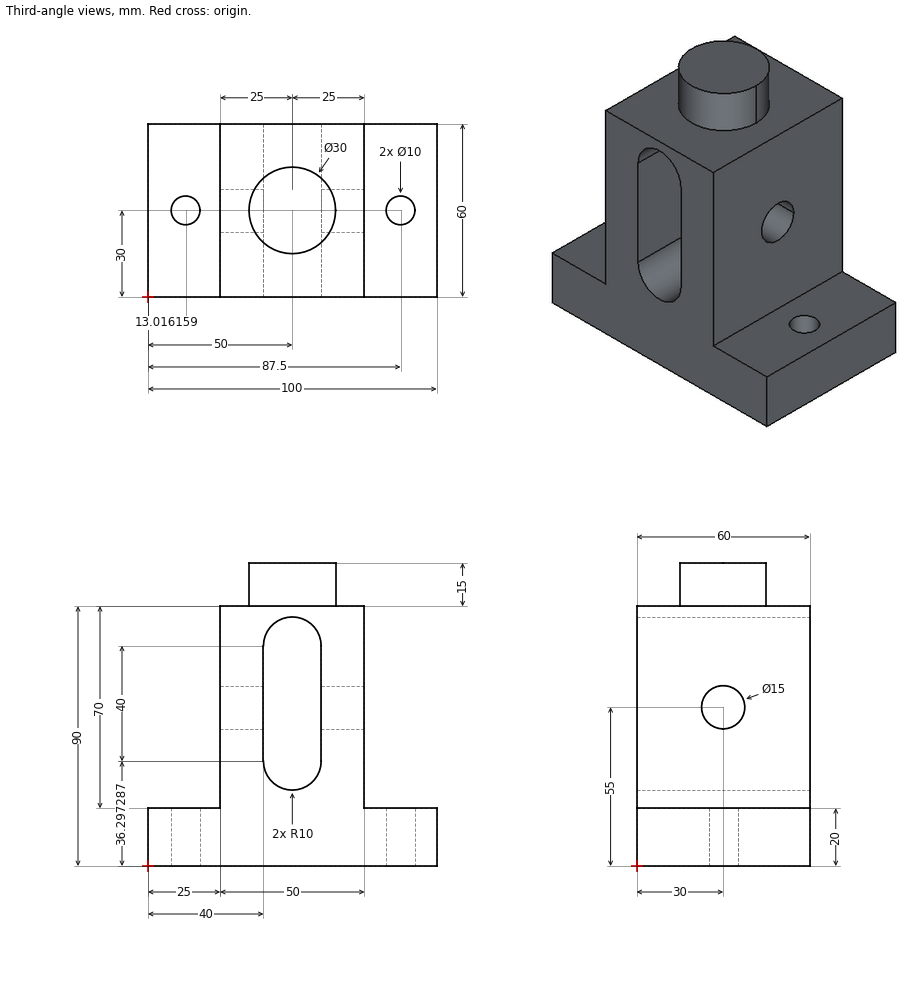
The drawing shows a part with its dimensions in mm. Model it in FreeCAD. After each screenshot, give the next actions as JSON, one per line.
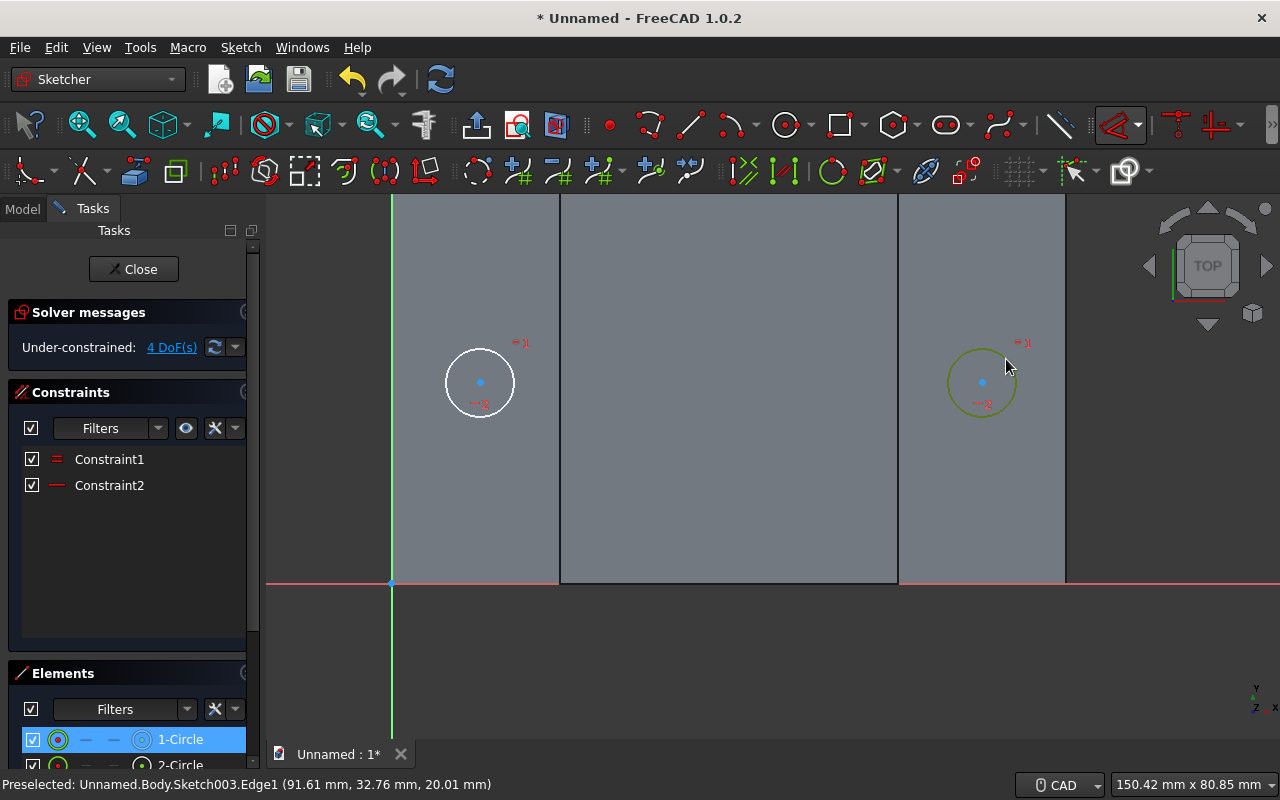
{"action": "left_click", "coordinate": [1140, 126]}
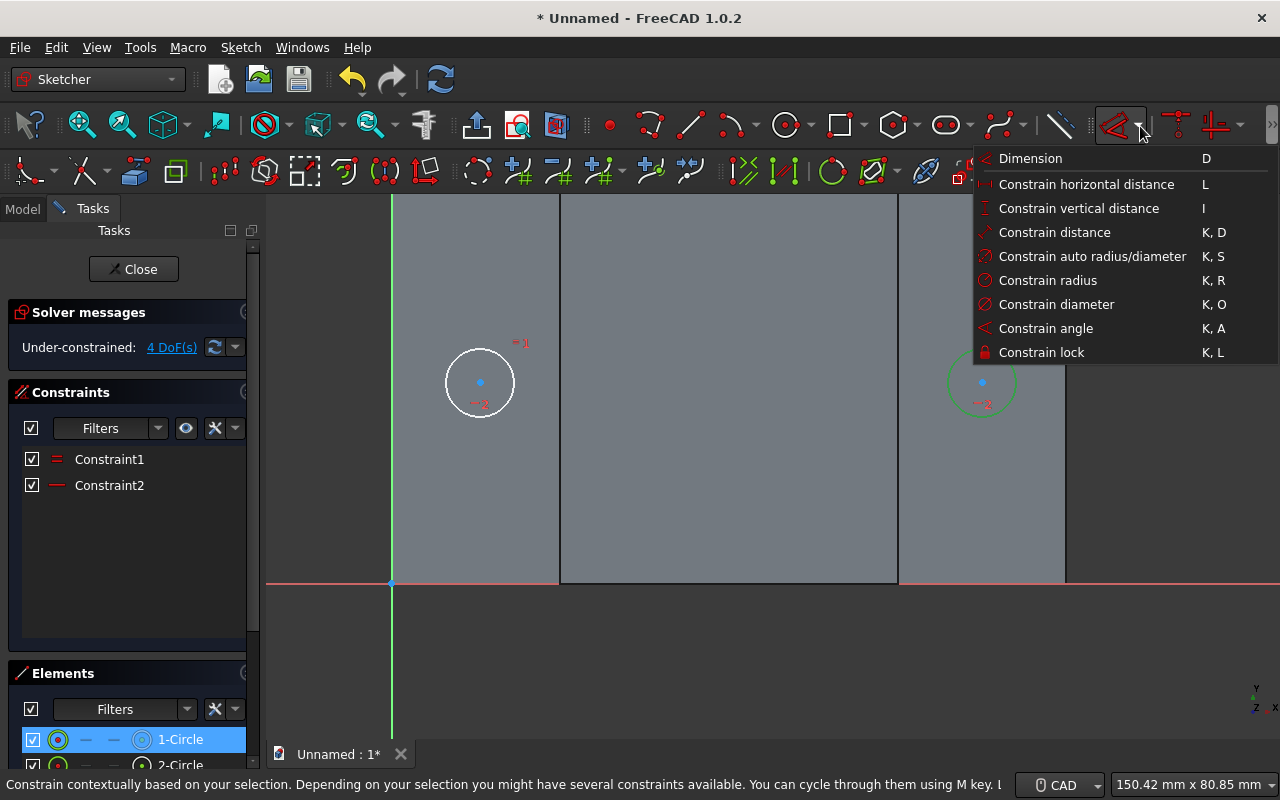
{"action": "left_click", "coordinate": [1126, 304]}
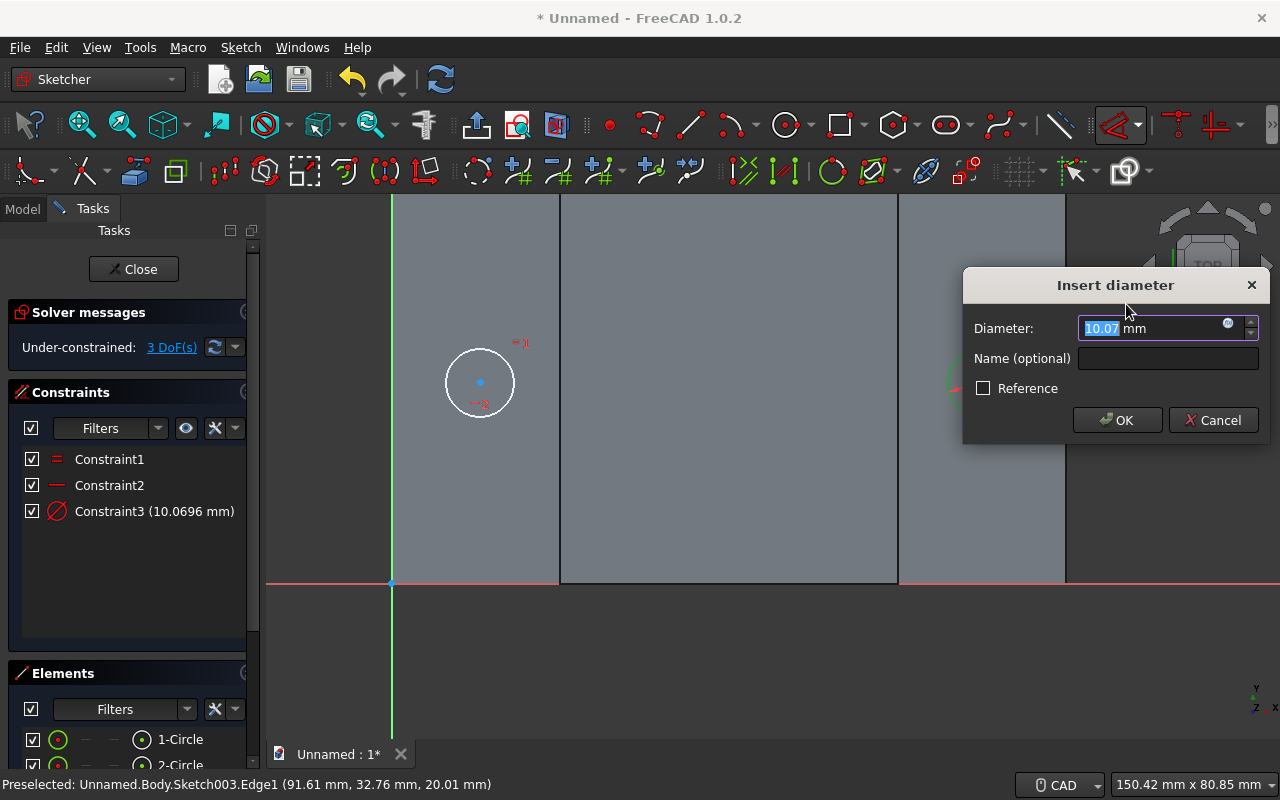
{"action": "type", "text": "10"}
{"action": "key", "text": "Return"}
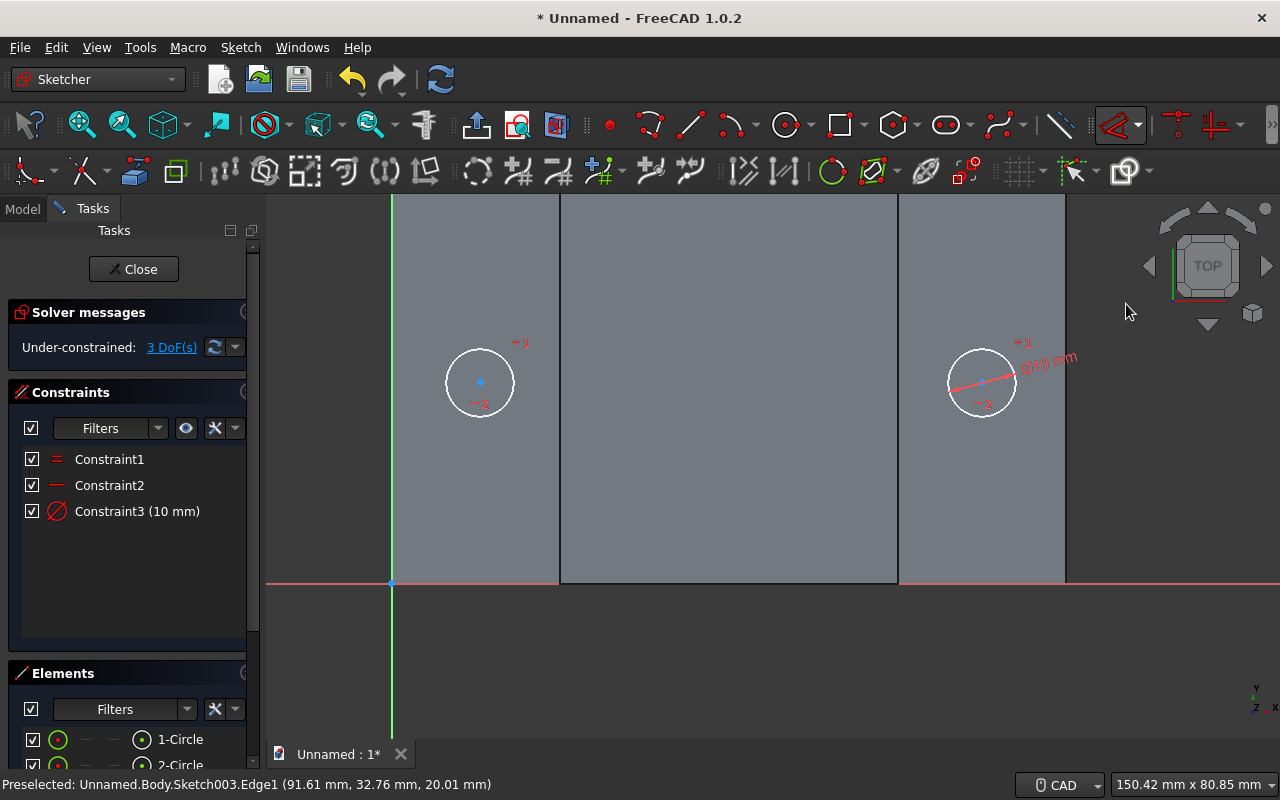
{"action": "left_click", "coordinate": [982, 383]}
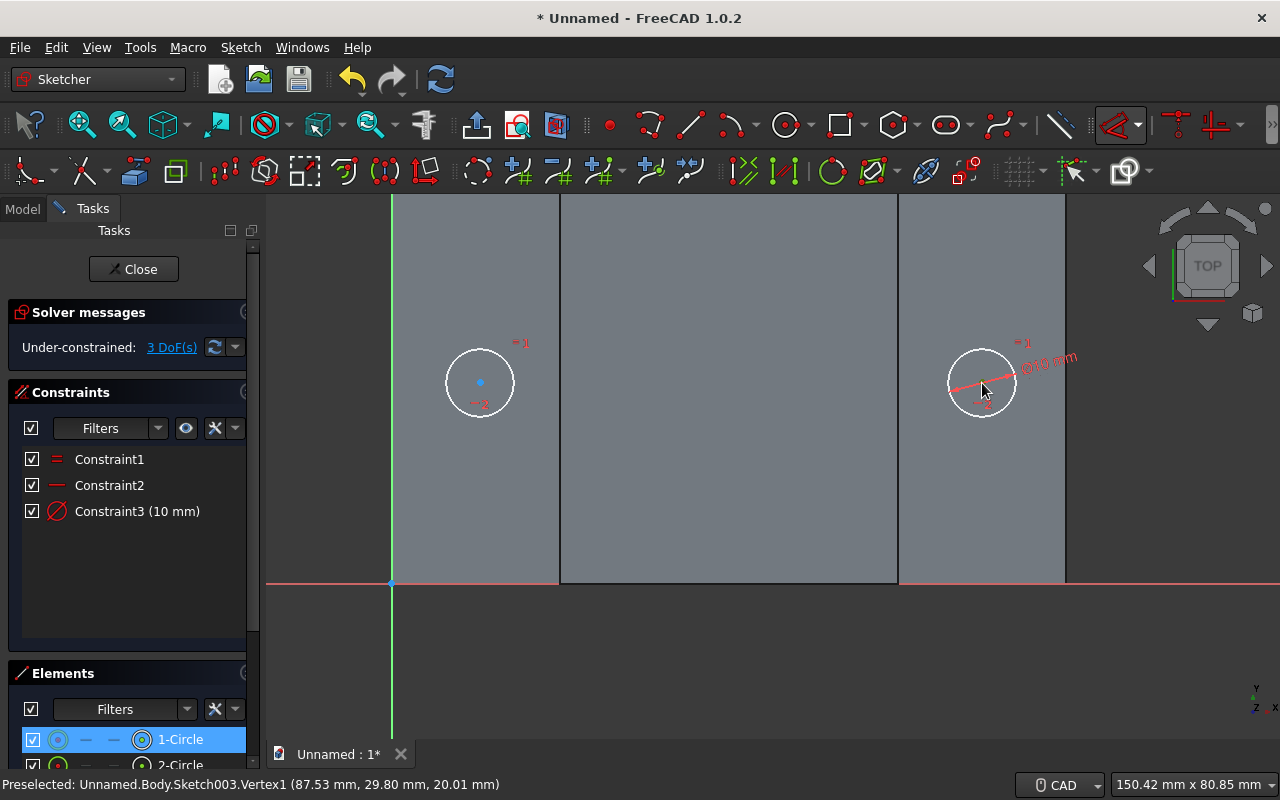
{"action": "key", "text": "i"}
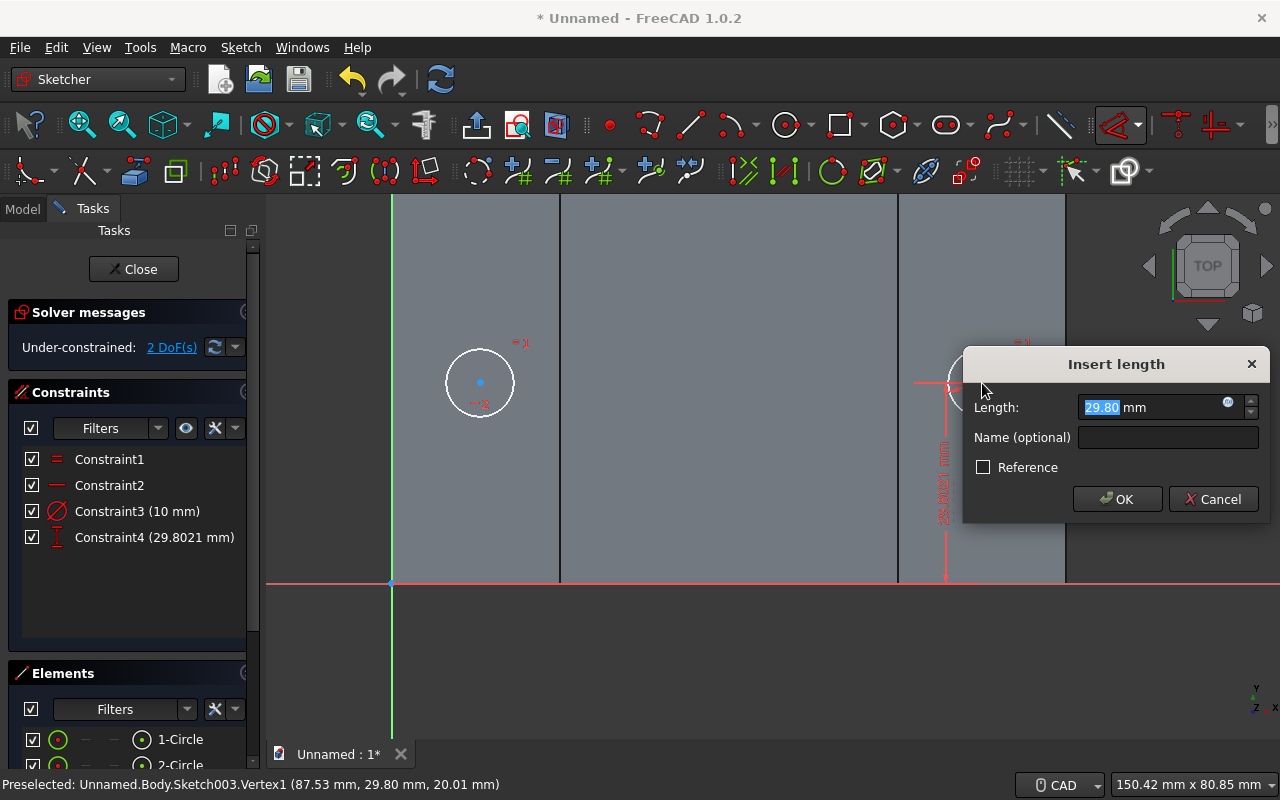
{"action": "type", "text": "30"}
{"action": "key", "text": "Return"}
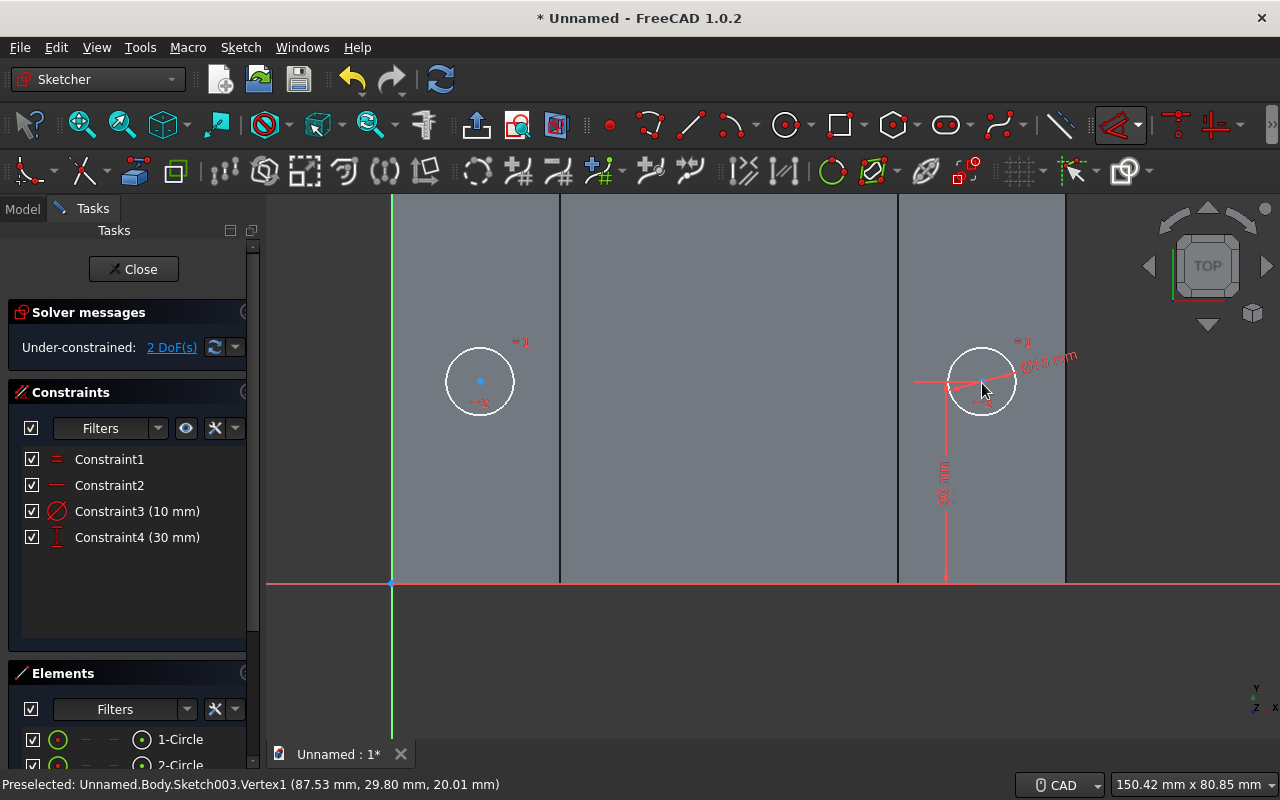
{"action": "left_click", "coordinate": [982, 382]}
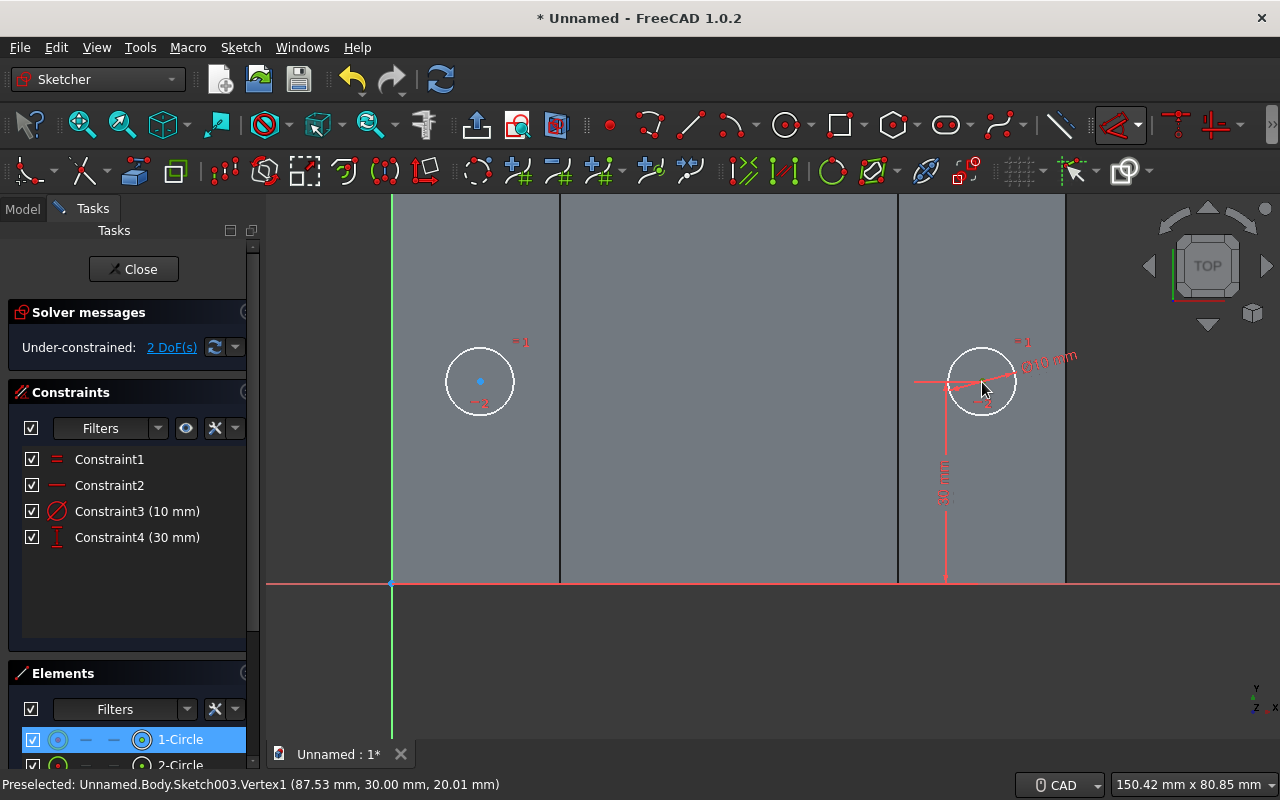
{"action": "key", "text": "l"}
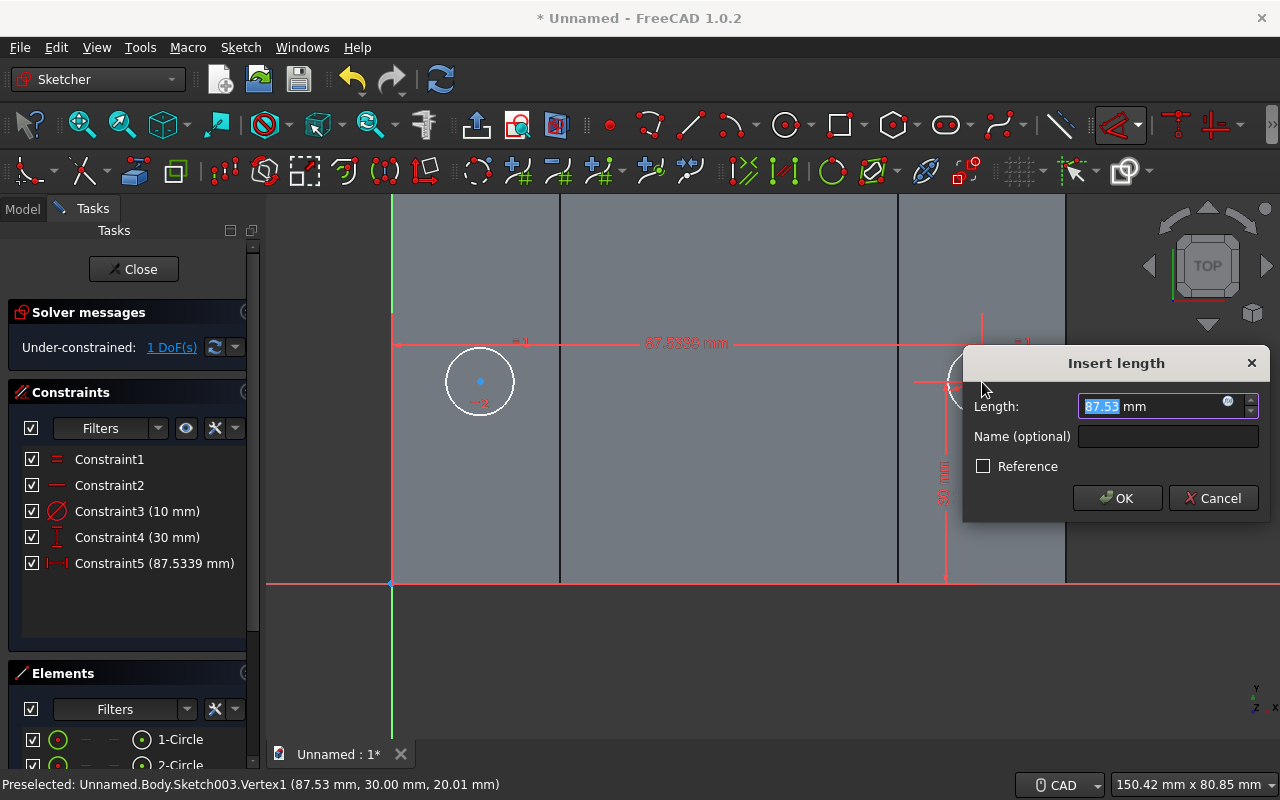
{"action": "type", "text": "87.5"}
{"action": "key", "text": "Return"}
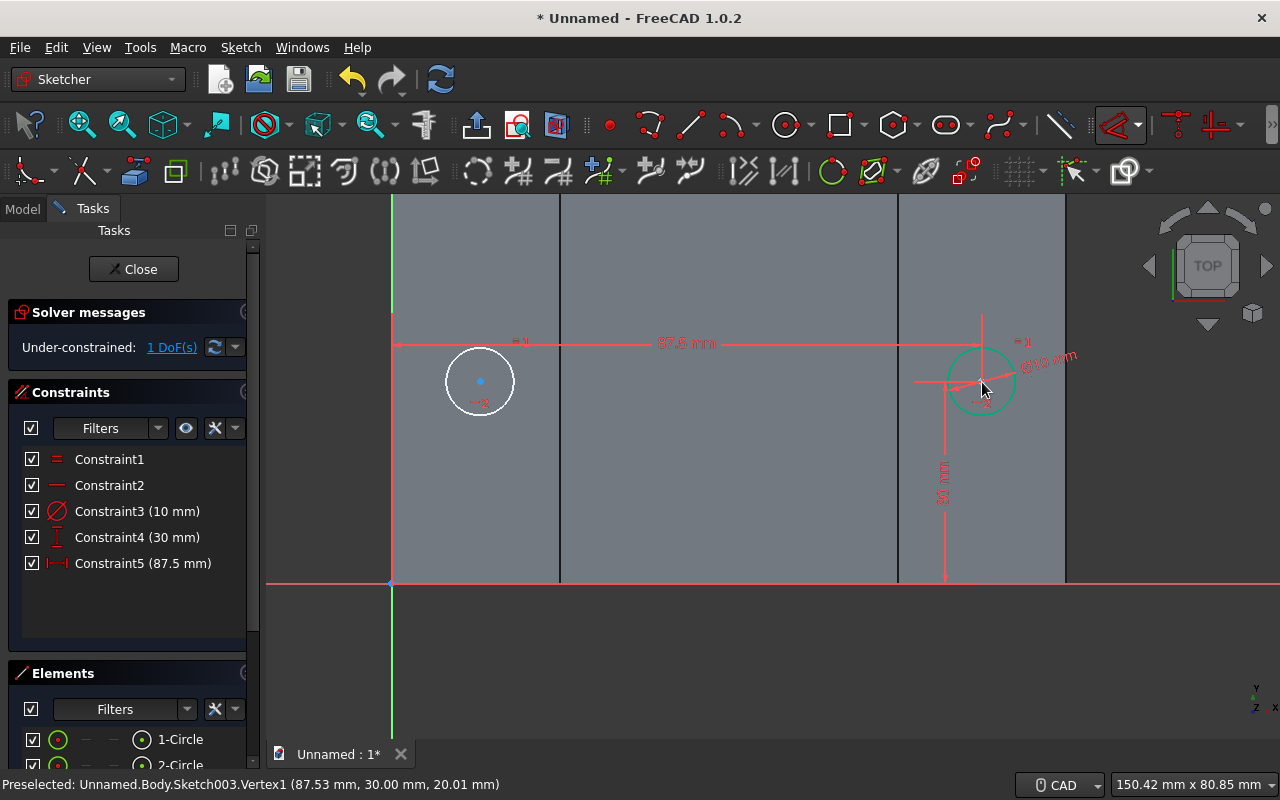
{"action": "left_click", "coordinate": [480, 382]}